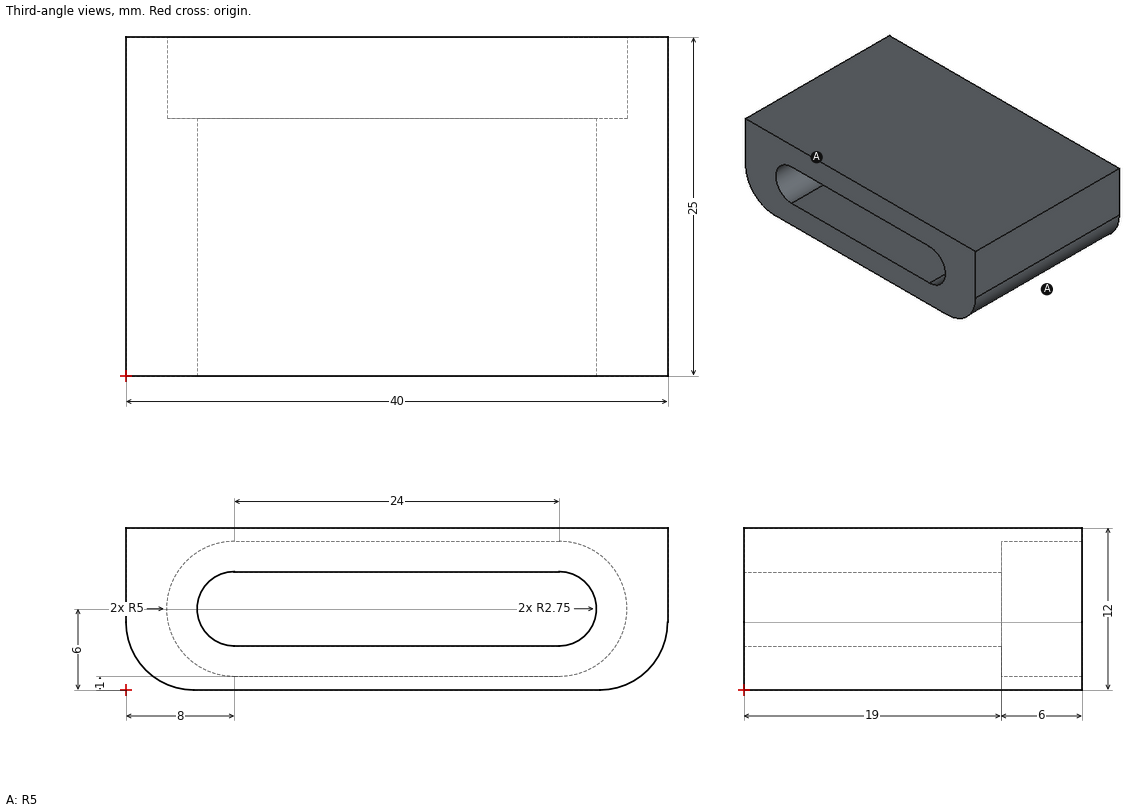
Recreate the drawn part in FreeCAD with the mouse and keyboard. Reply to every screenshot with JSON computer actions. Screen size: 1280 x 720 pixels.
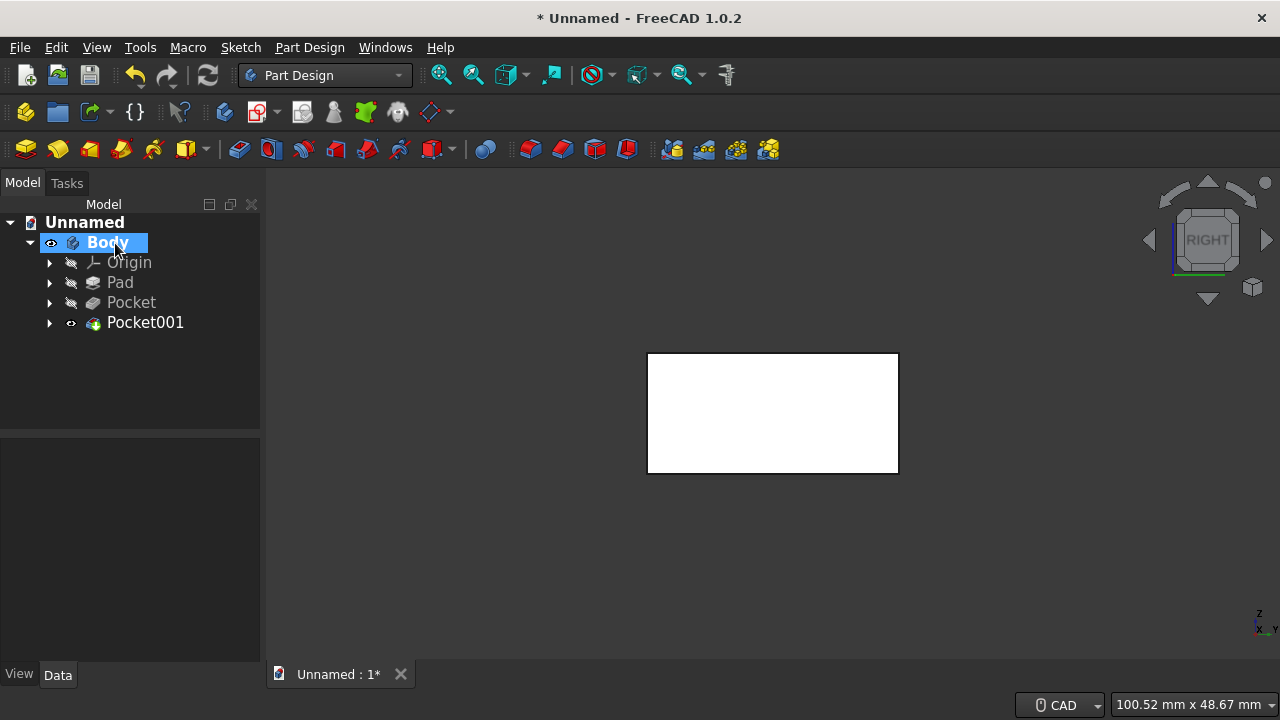
{"action": "left_click", "coordinate": [773, 473]}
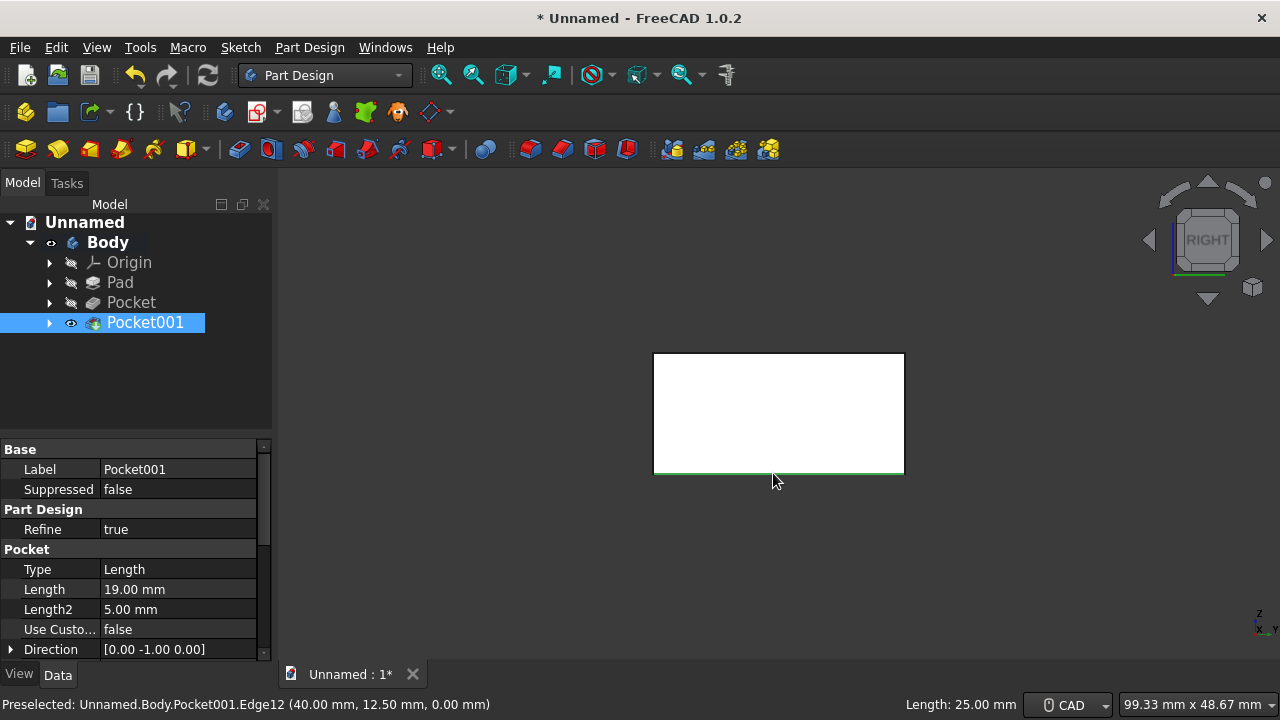
{"action": "key", "text": "5"}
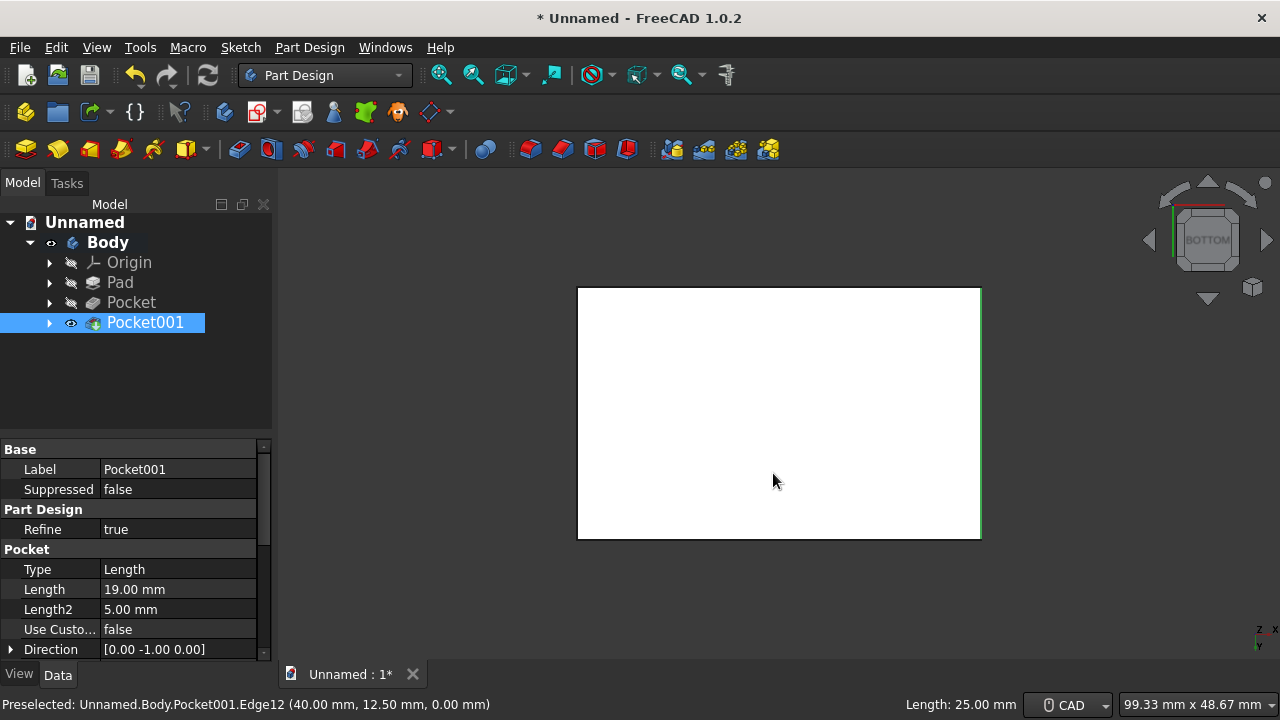
{"action": "left_click", "coordinate": [577, 412], "text": "ctrl"}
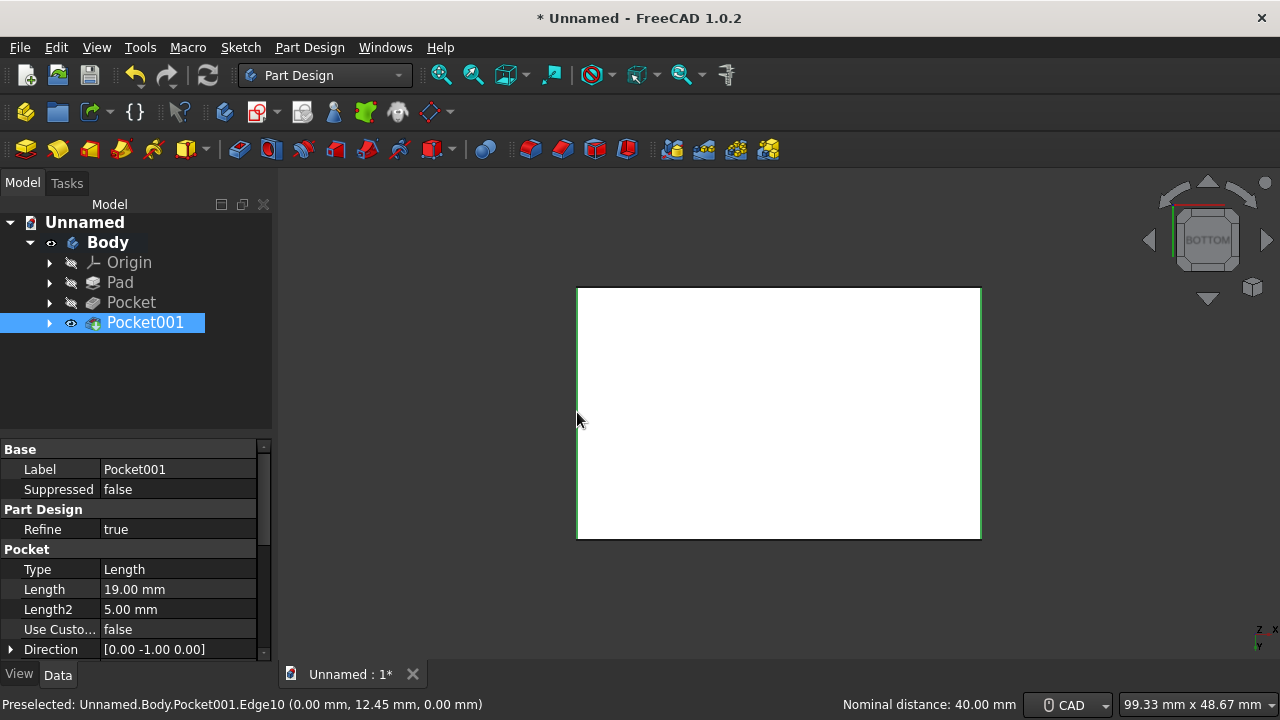
{"action": "left_click", "coordinate": [532, 150]}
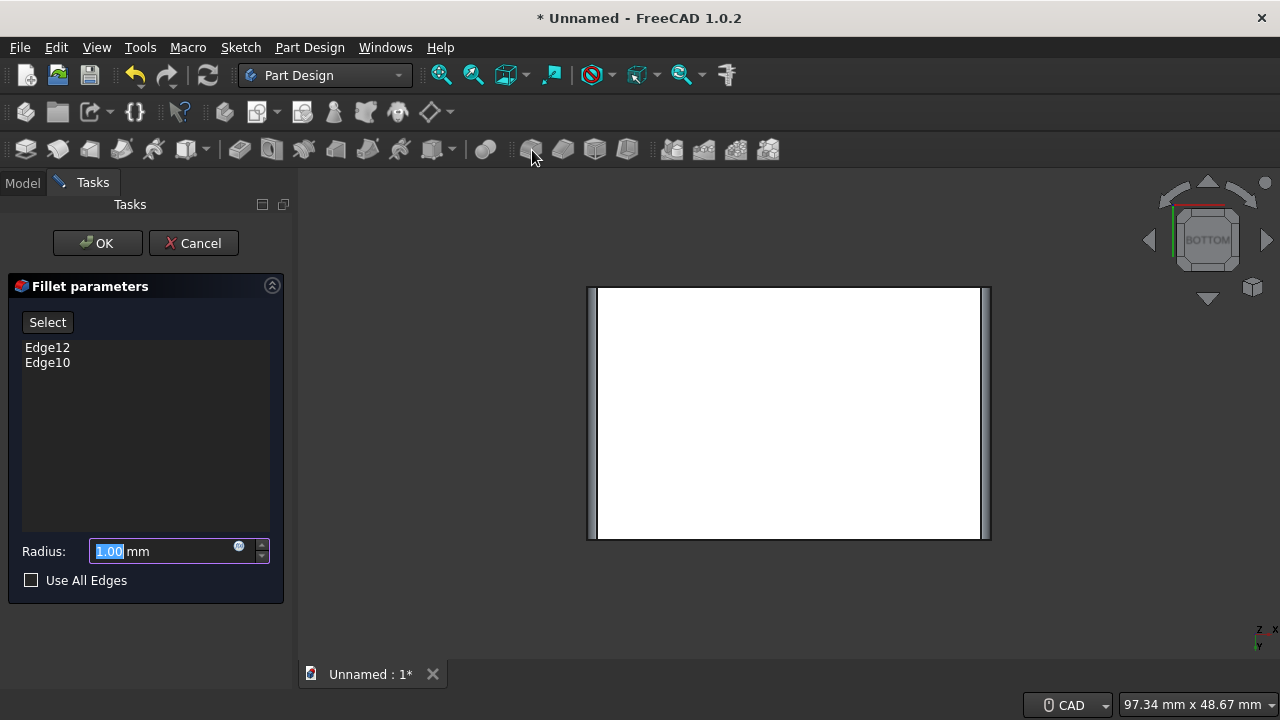
{"action": "type", "text": "5"}
{"action": "key", "text": "Tab"}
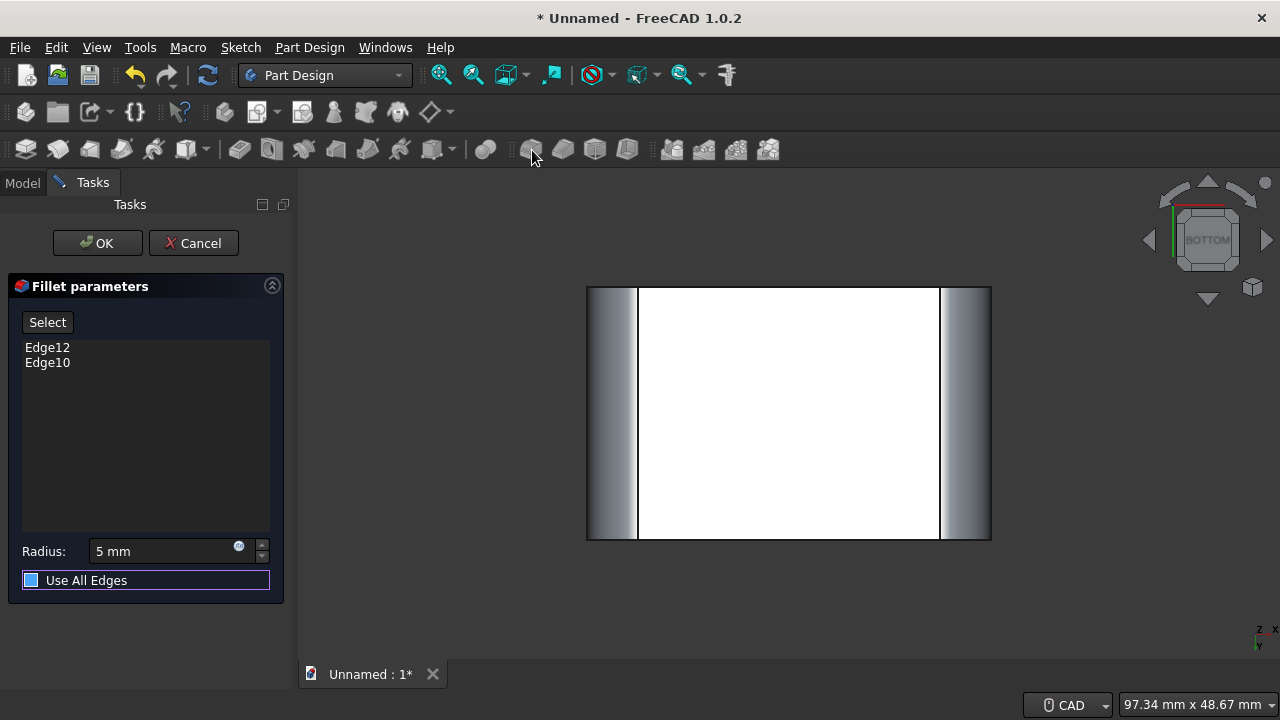
{"action": "left_click", "coordinate": [98, 243]}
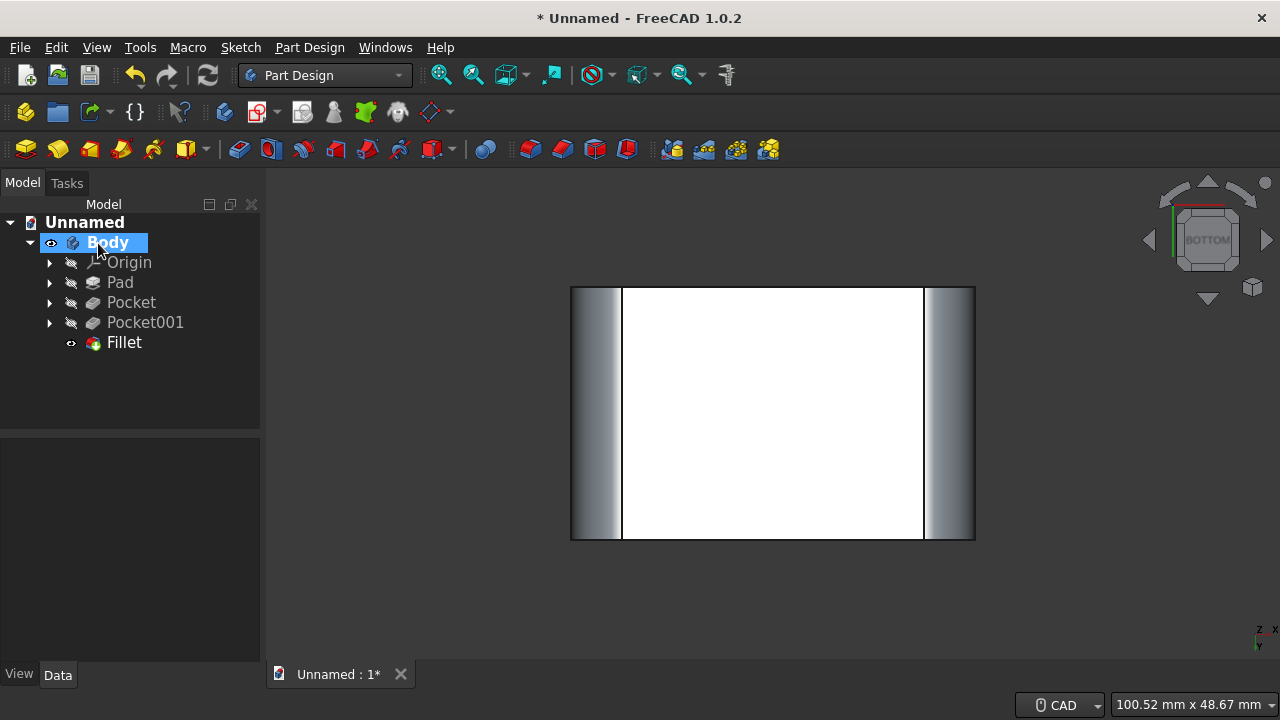
{"action": "key", "text": "0"}